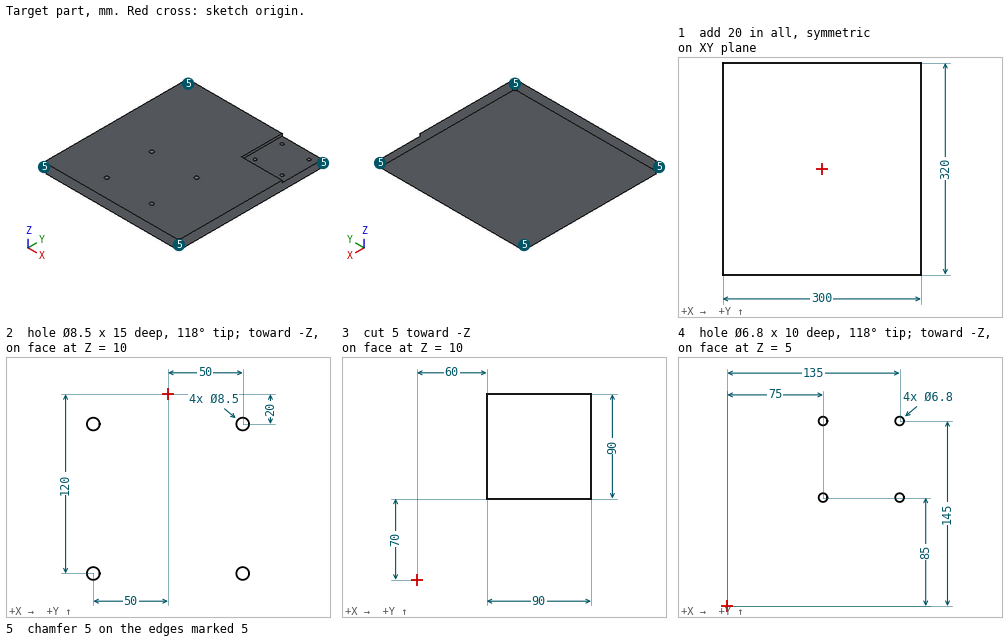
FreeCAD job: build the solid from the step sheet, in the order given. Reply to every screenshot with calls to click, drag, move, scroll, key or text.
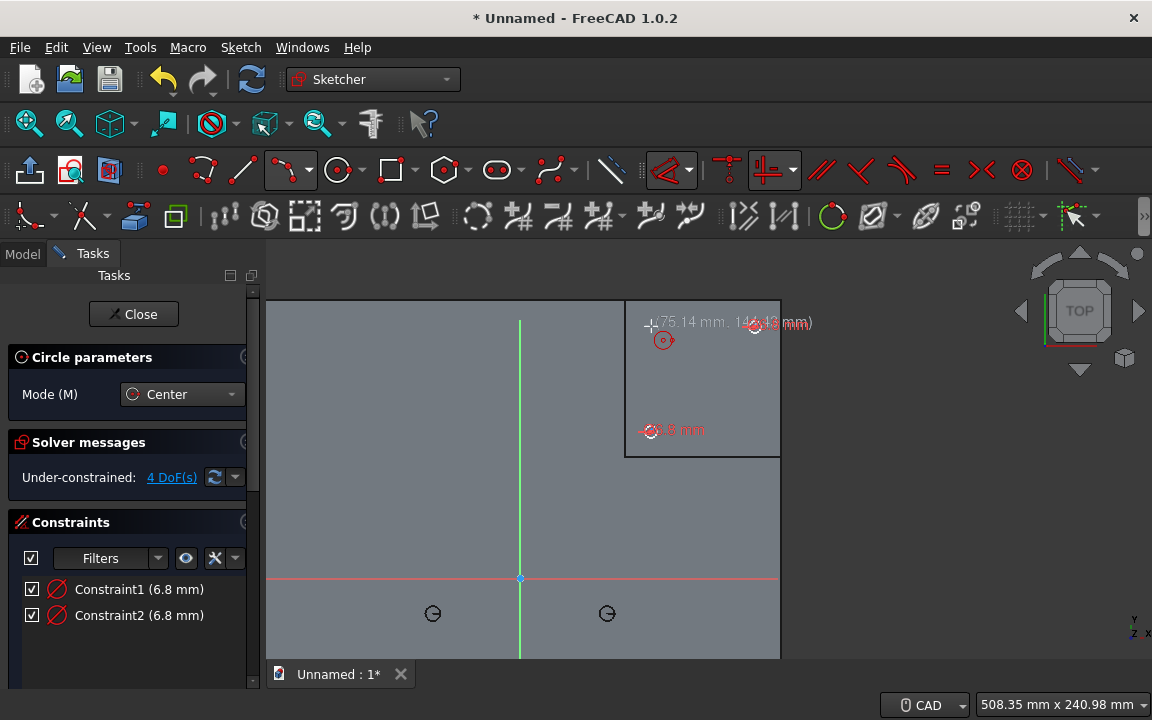
click(651, 326)
move(655, 322)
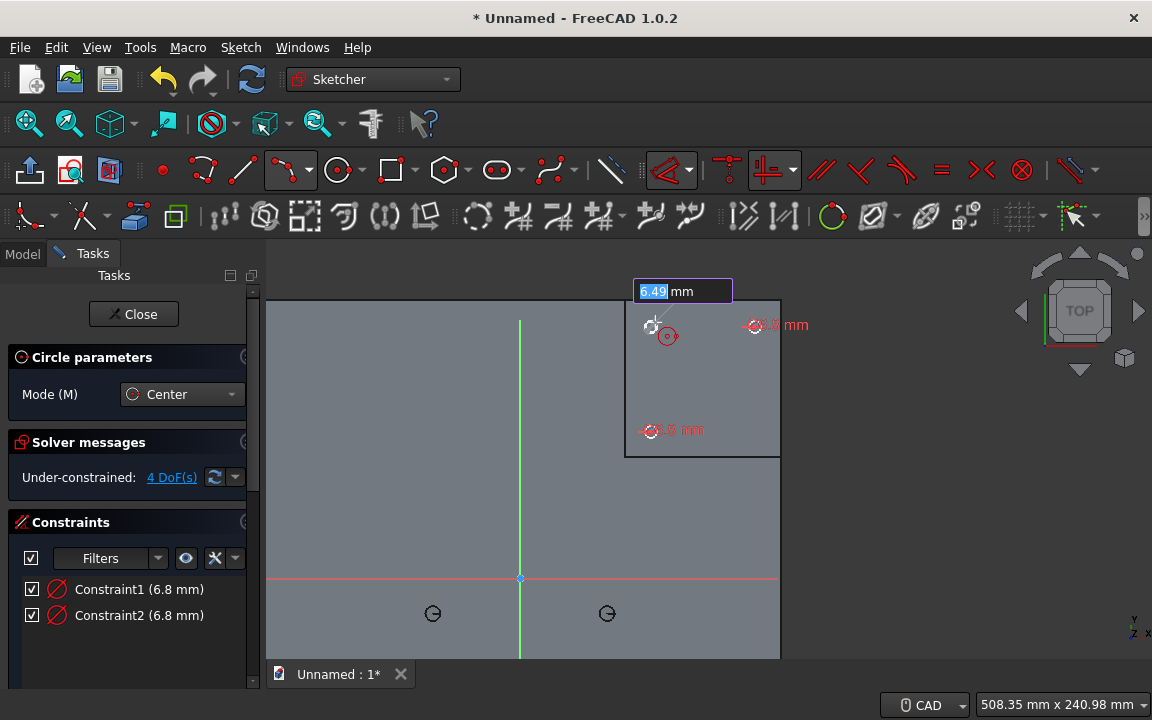
text(6.8)
key(Return)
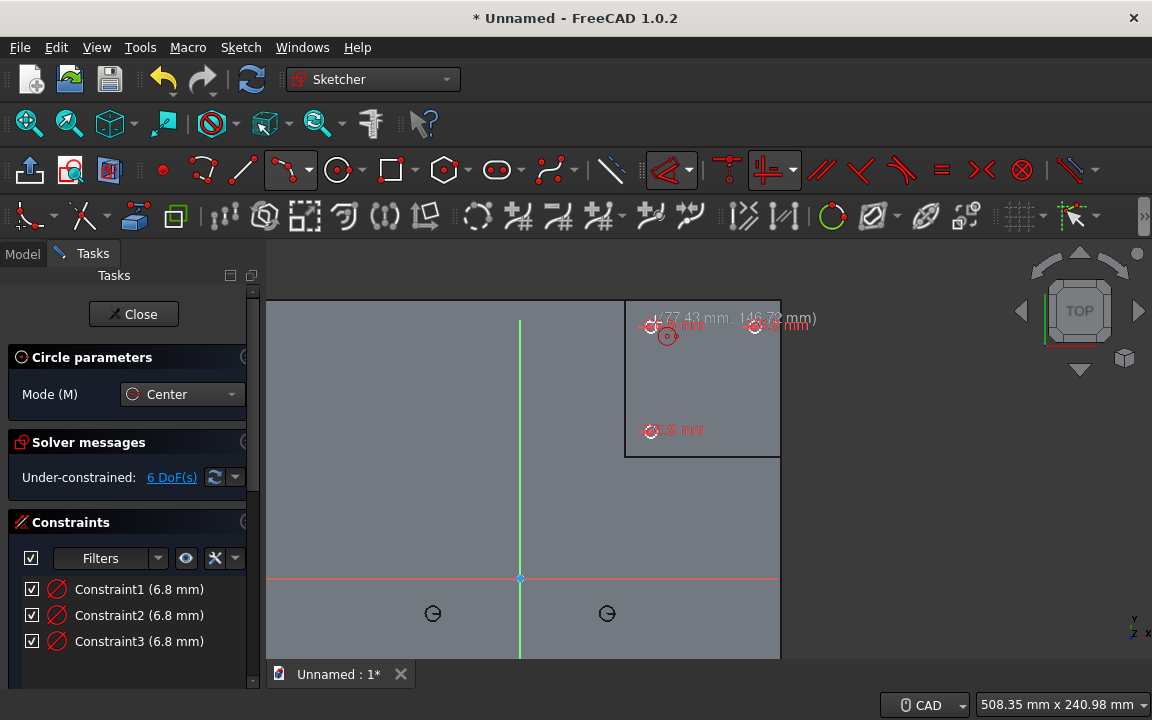
scroll(755, 431, up, 7)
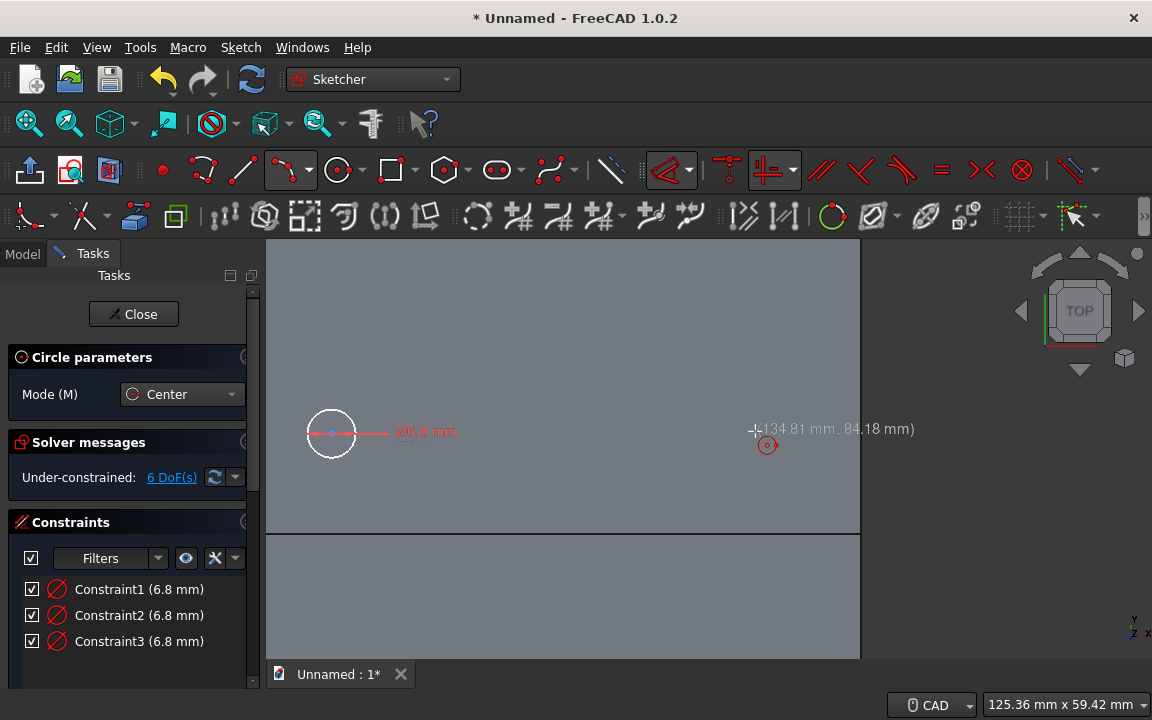
scroll(755, 431, down, 7)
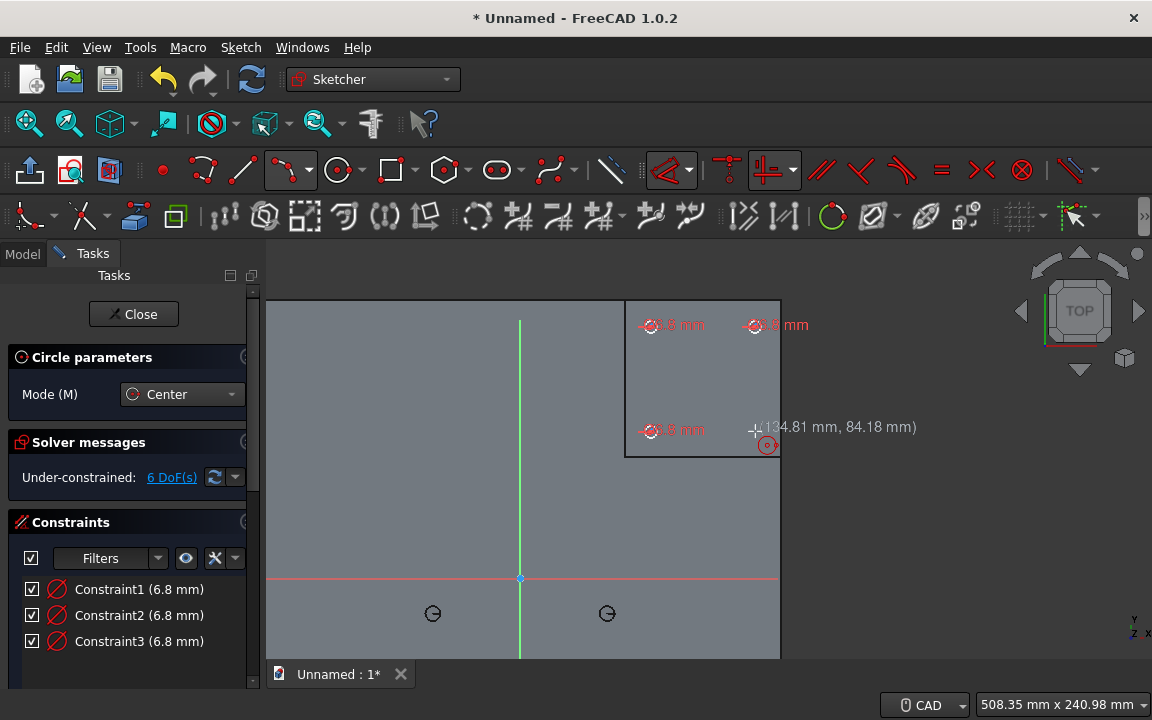
click(755, 431)
move(760, 426)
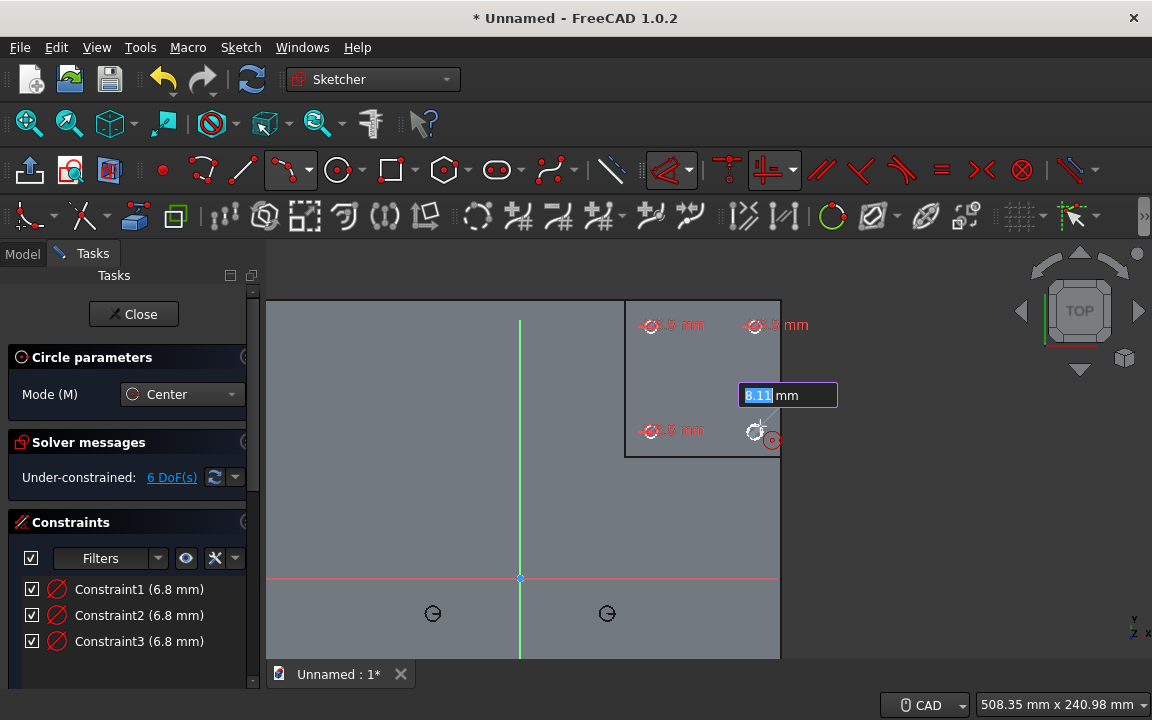
text(6.8)
key(Return)
key(Escape)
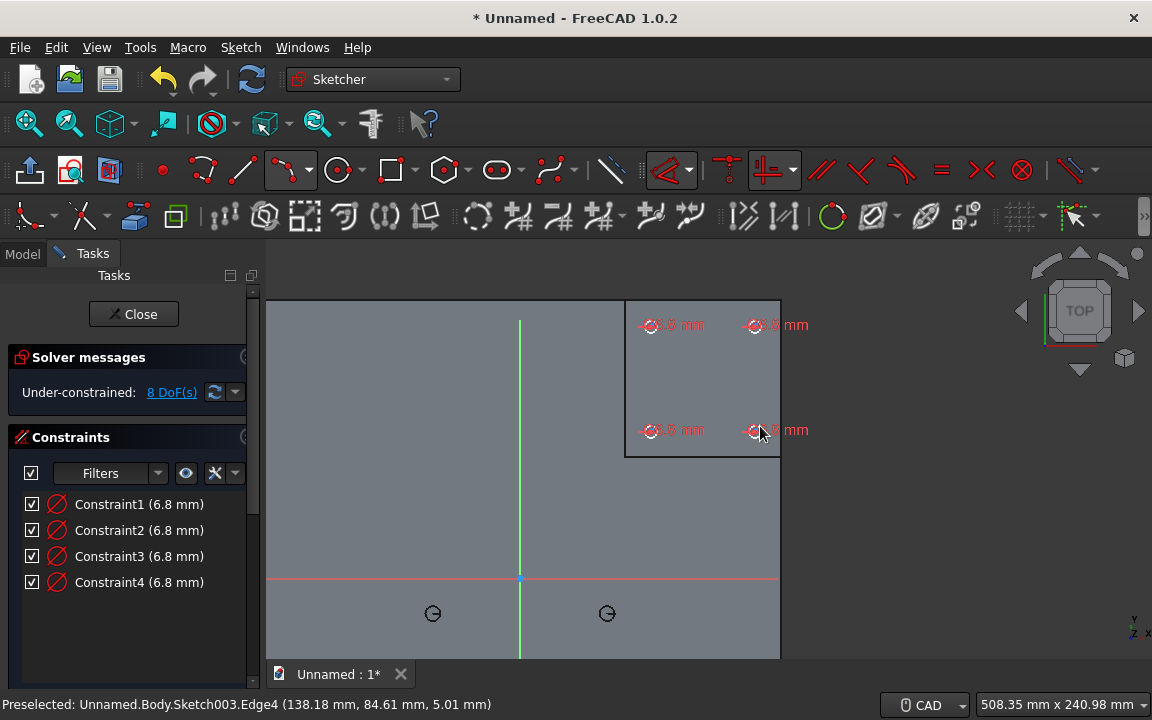
click(651, 432)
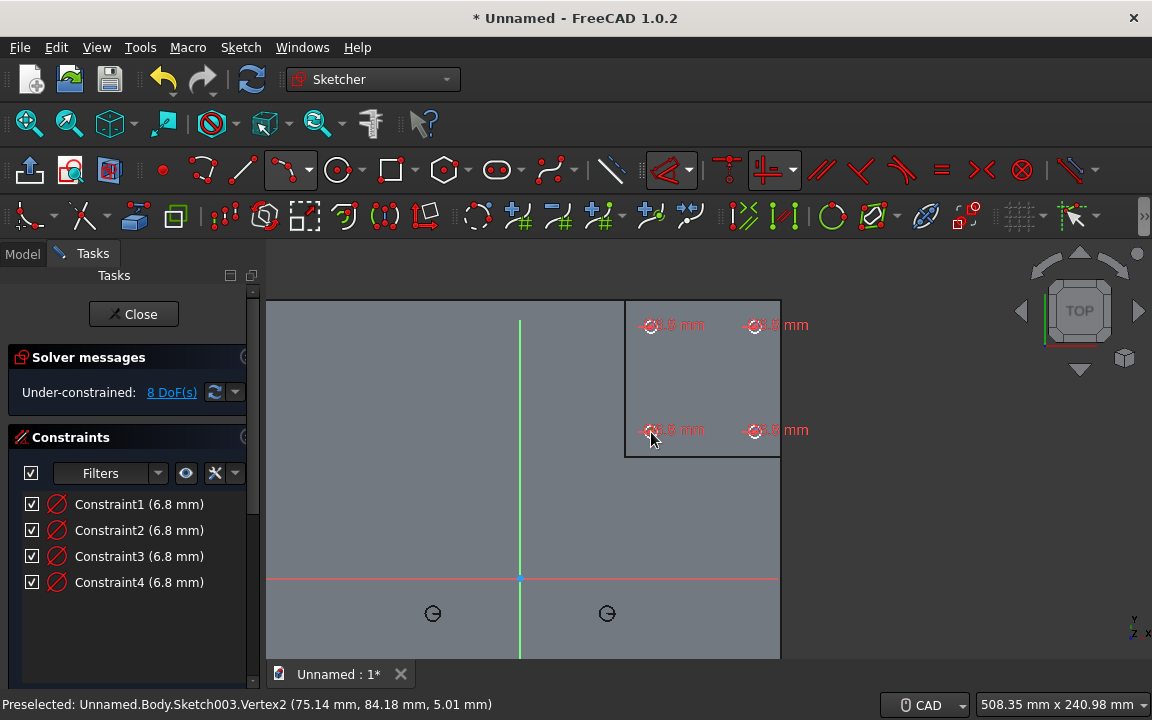
click(651, 327)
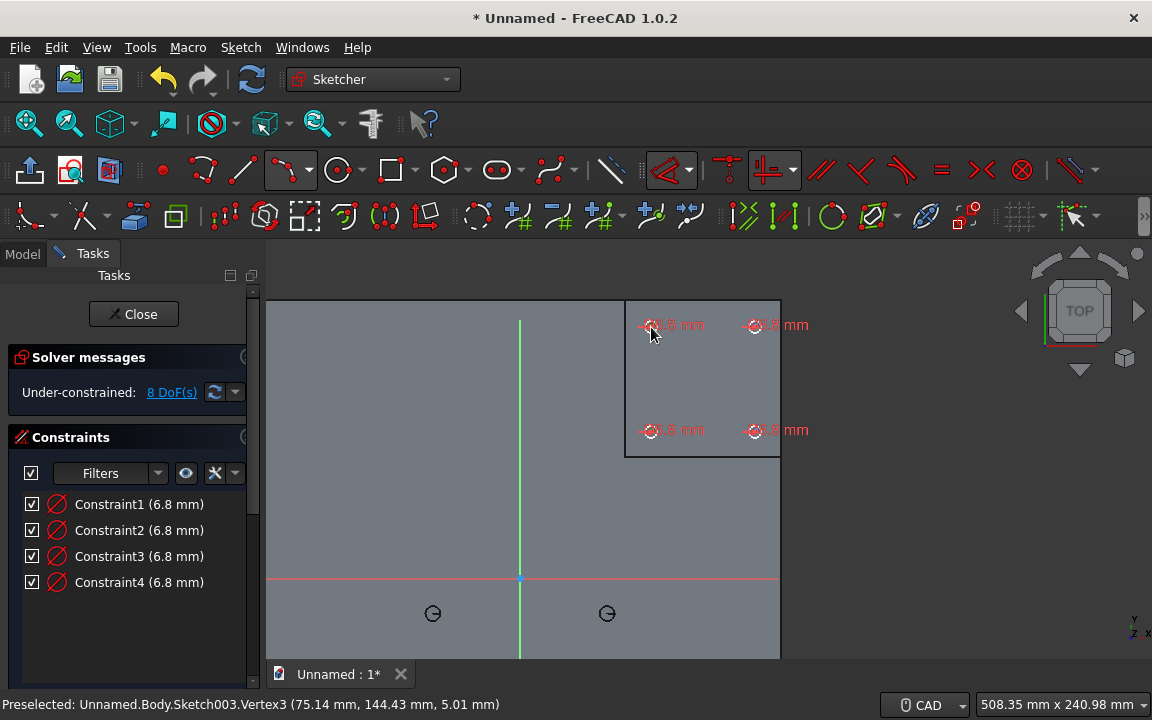
key(v)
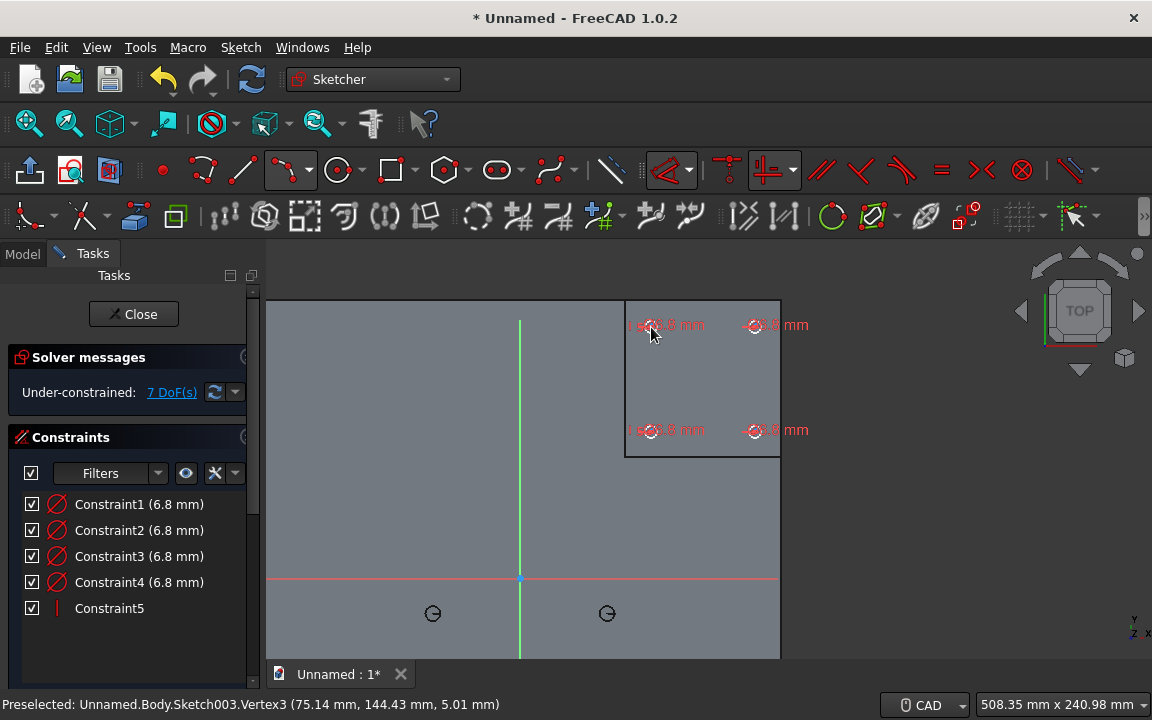
click(755, 327)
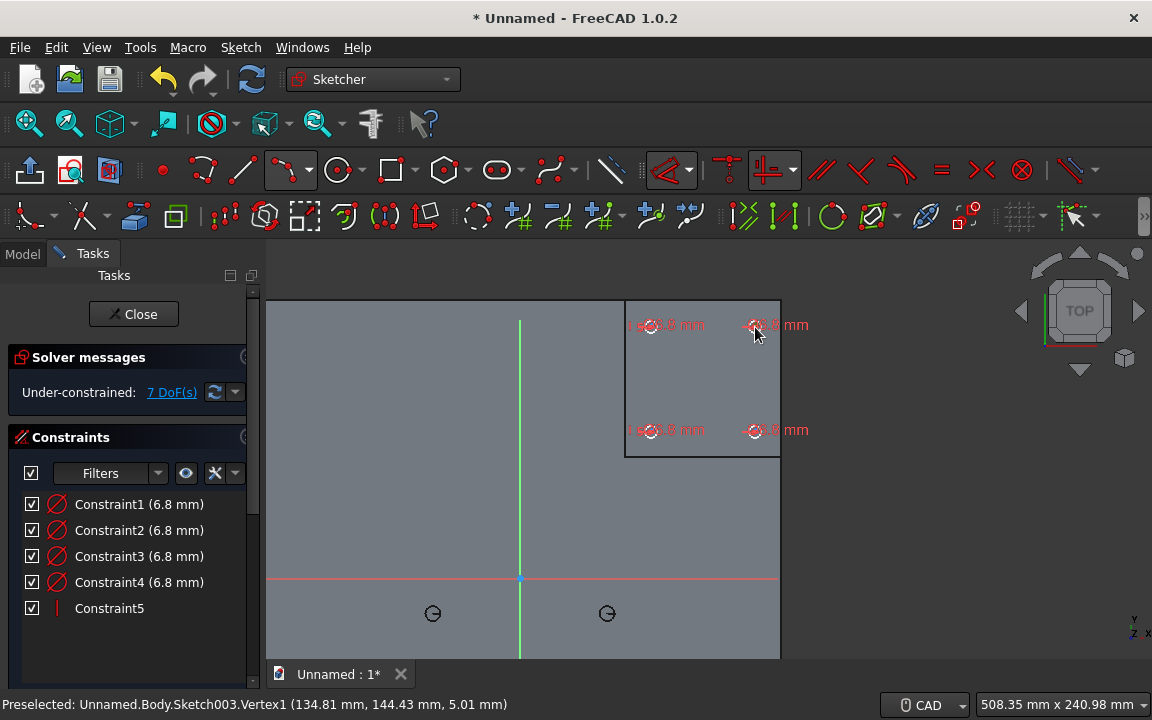
click(651, 327)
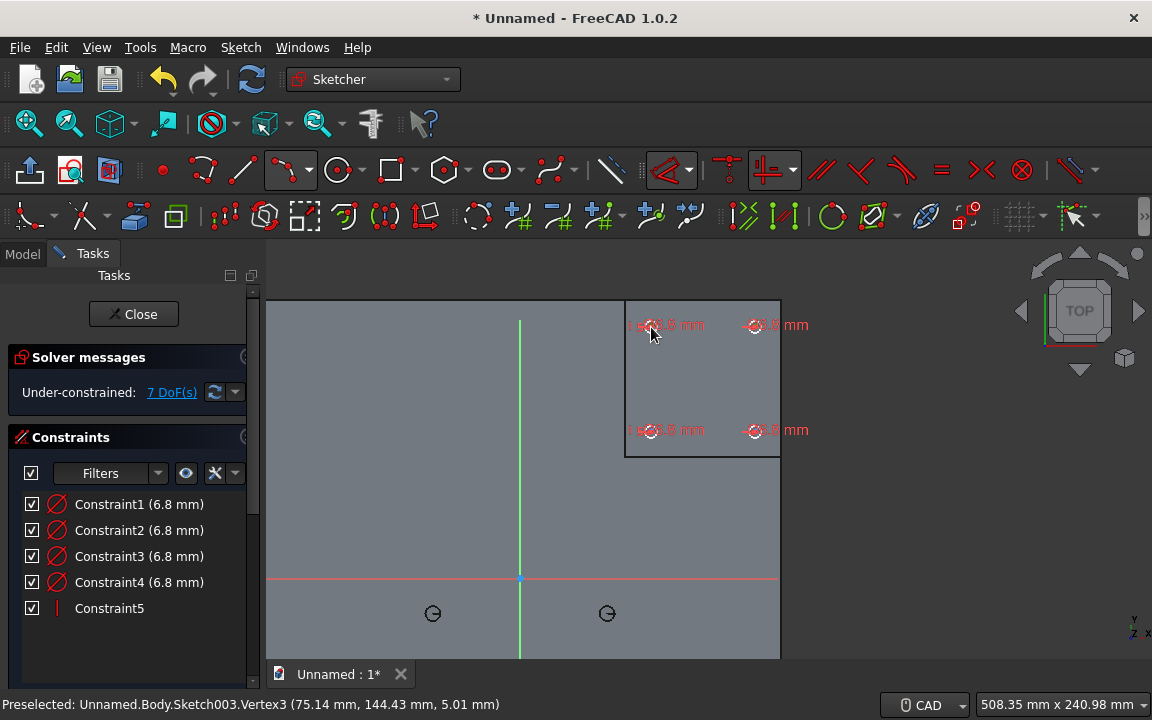
click(796, 170)